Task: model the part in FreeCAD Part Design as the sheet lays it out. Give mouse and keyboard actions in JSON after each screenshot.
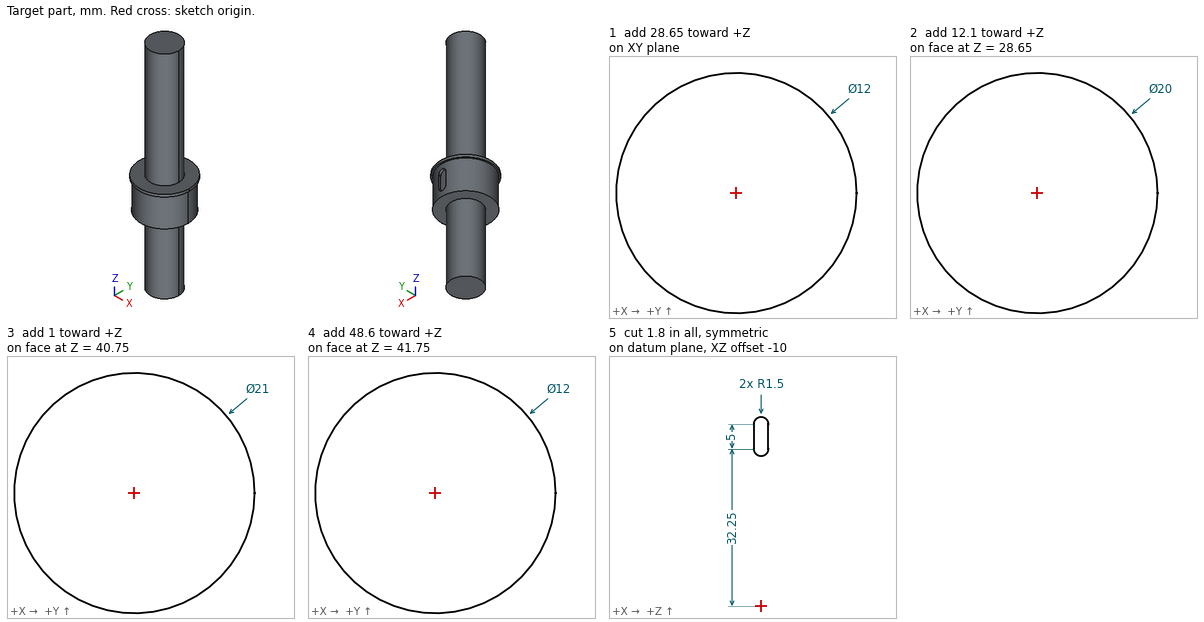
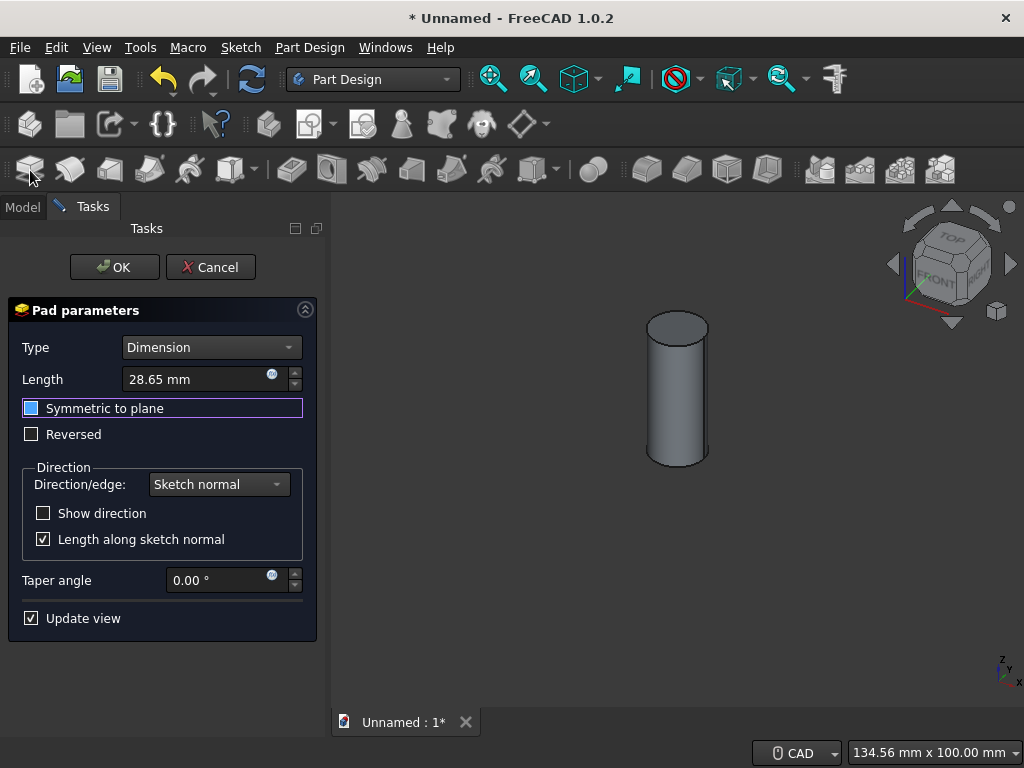
{"action": "left_click", "coordinate": [115, 267]}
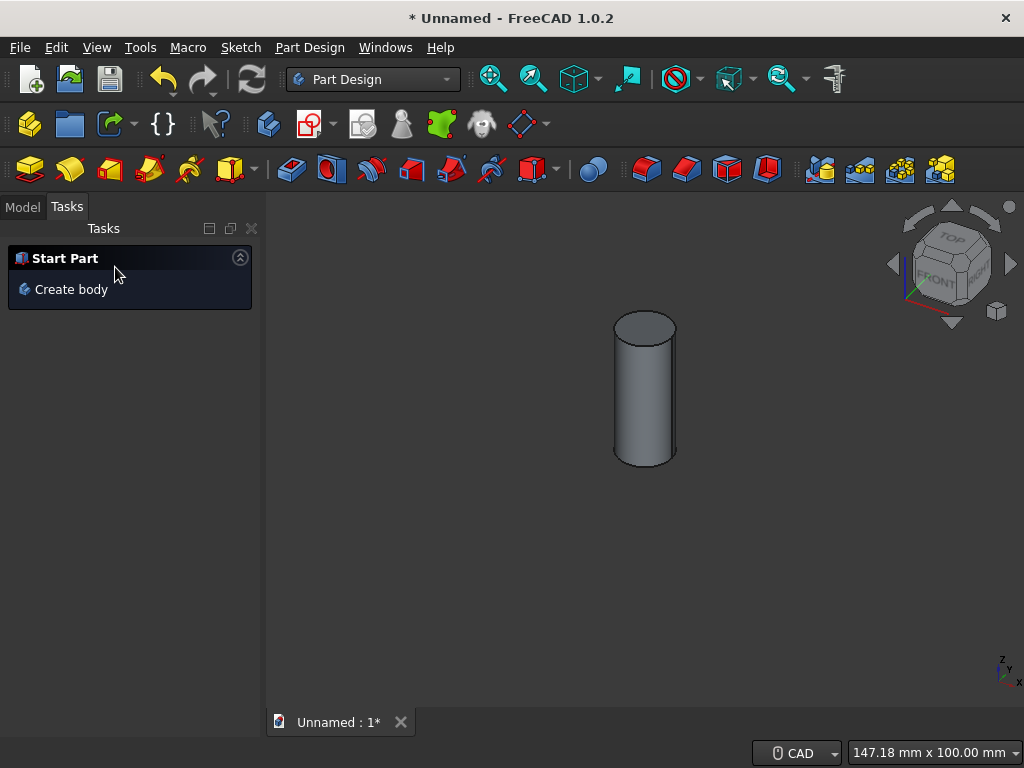
{"action": "left_click", "coordinate": [494, 80]}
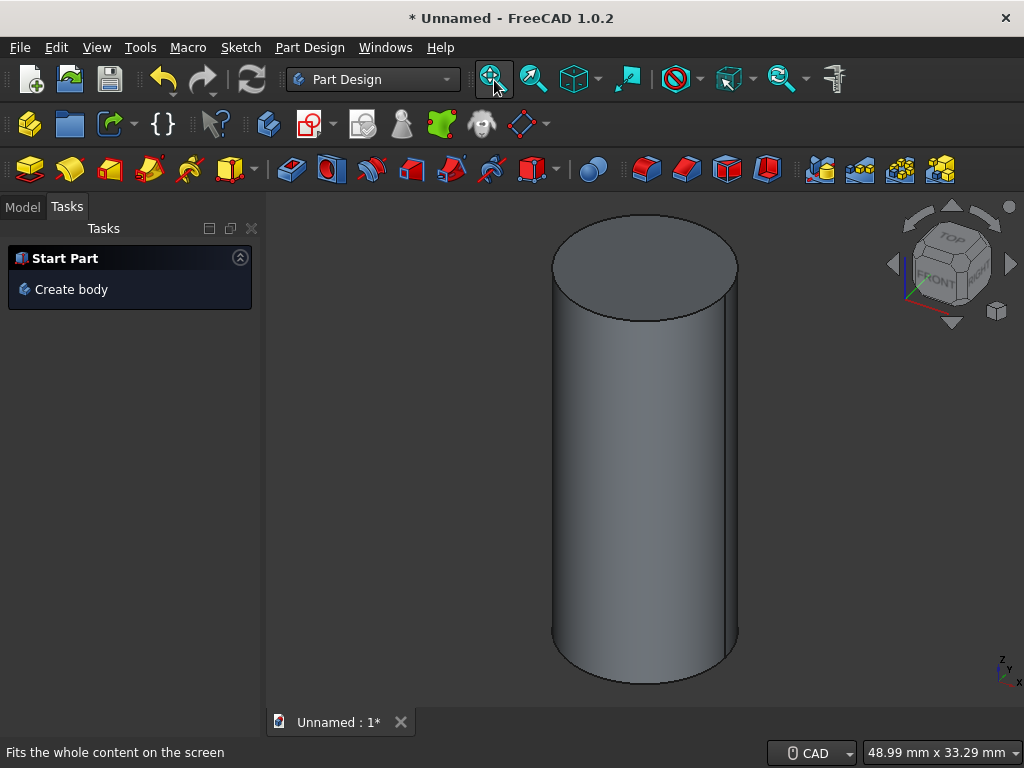
{"action": "left_click", "coordinate": [645, 267]}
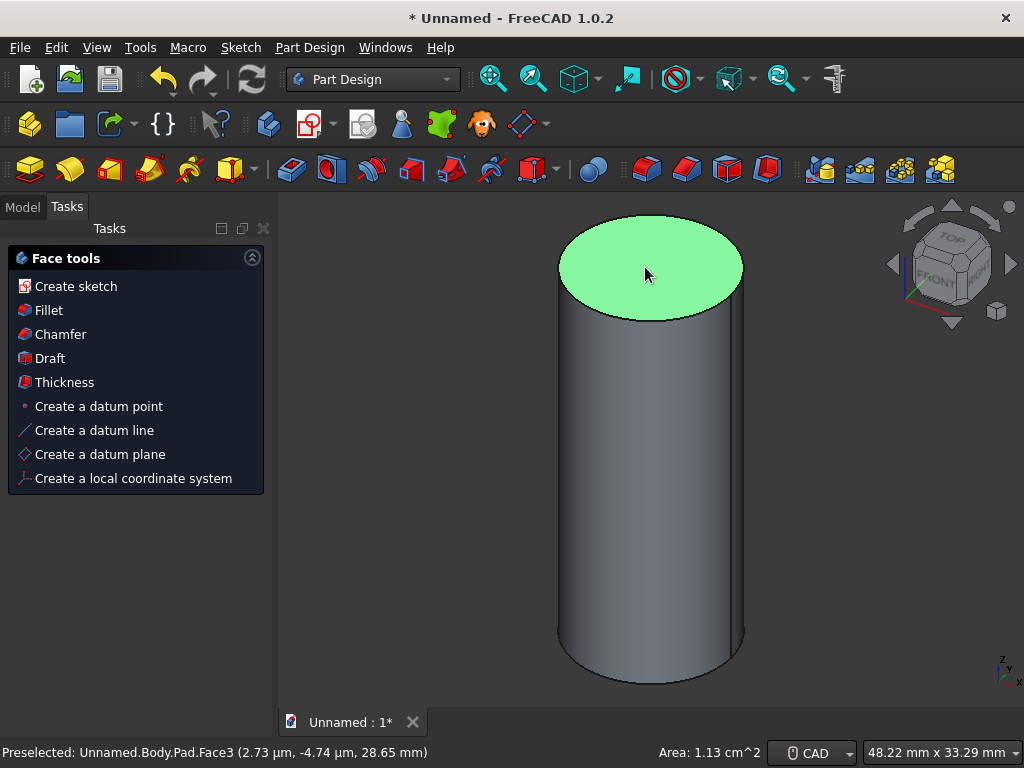
{"action": "left_click", "coordinate": [310, 124]}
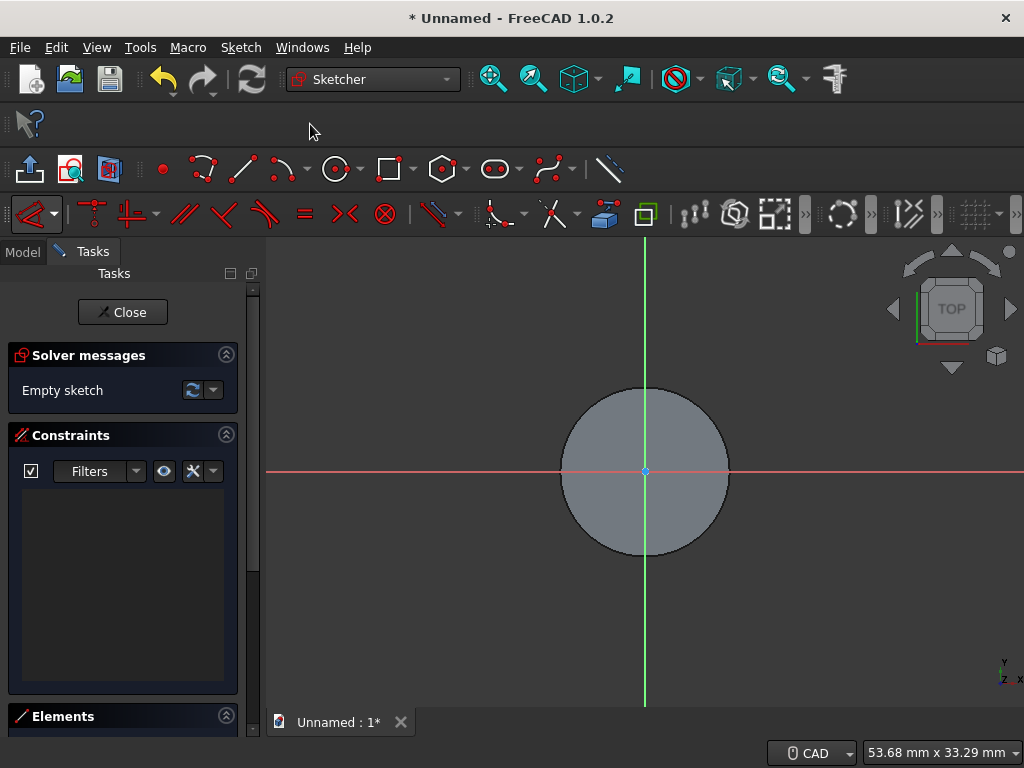
{"action": "left_click", "coordinate": [336, 170]}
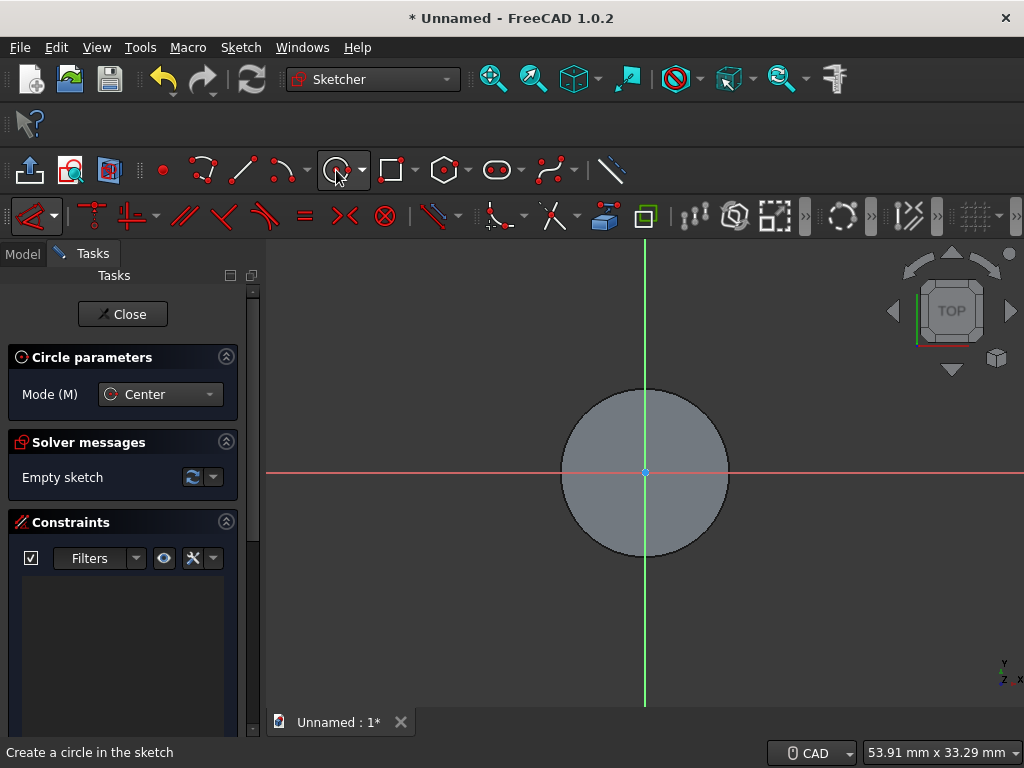
{"action": "left_click", "coordinate": [645, 473]}
{"action": "left_click", "coordinate": [744, 374]}
{"action": "key", "text": "Escape"}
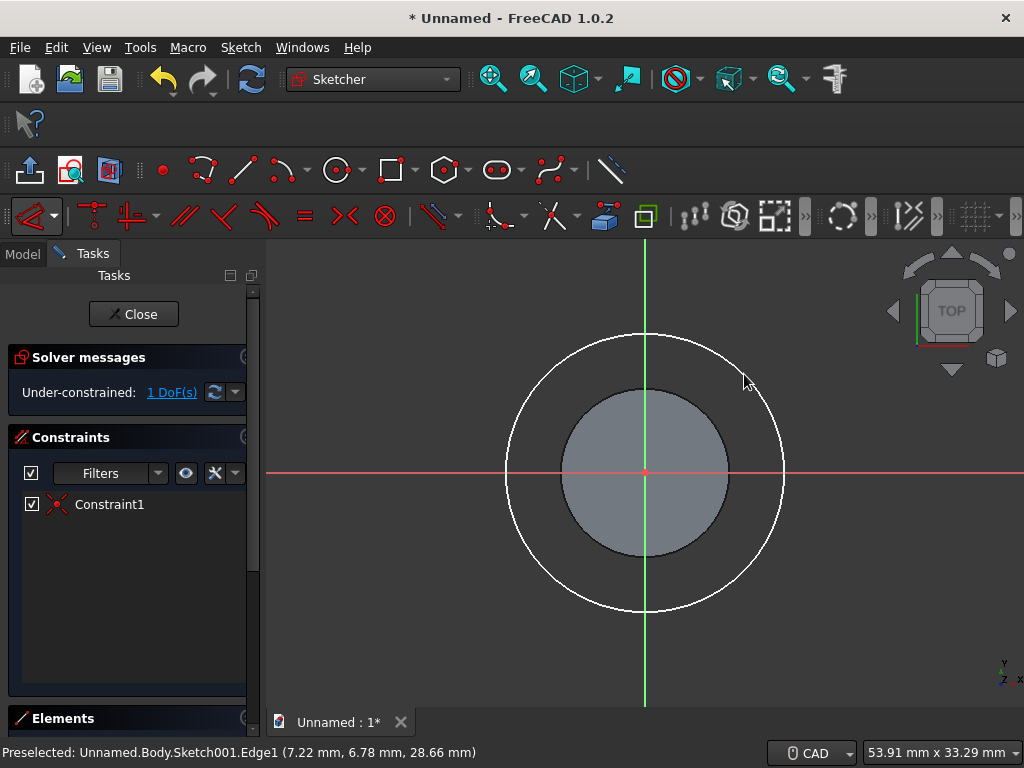
{"action": "left_click", "coordinate": [743, 374]}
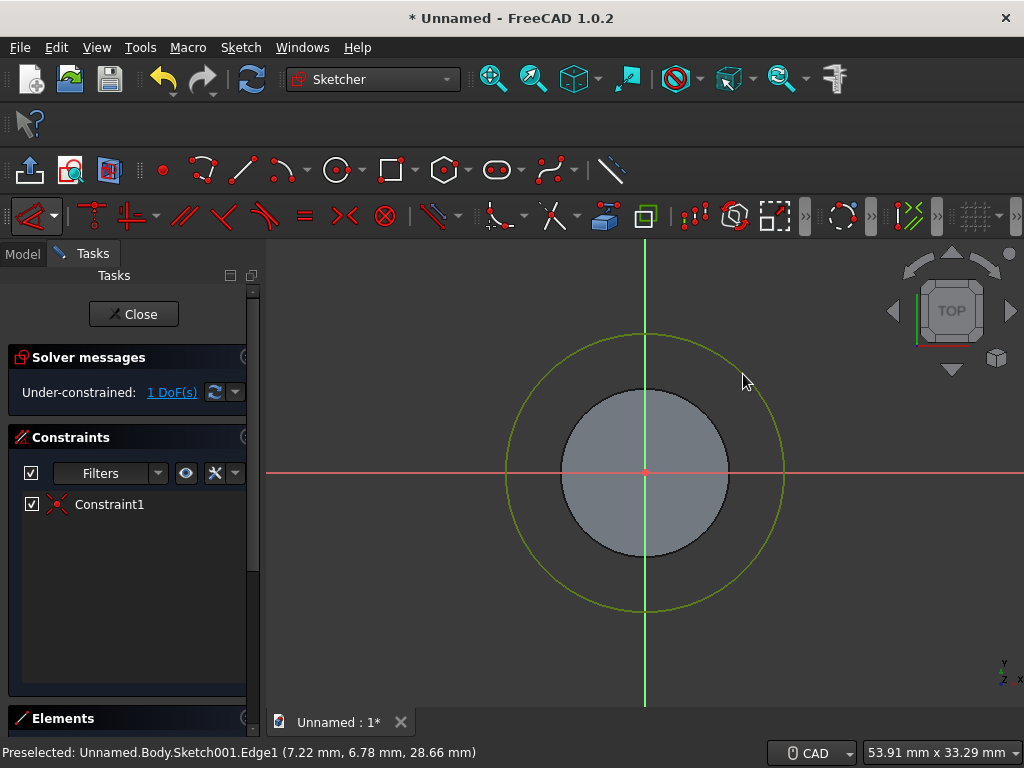
{"action": "left_click", "coordinate": [56, 216]}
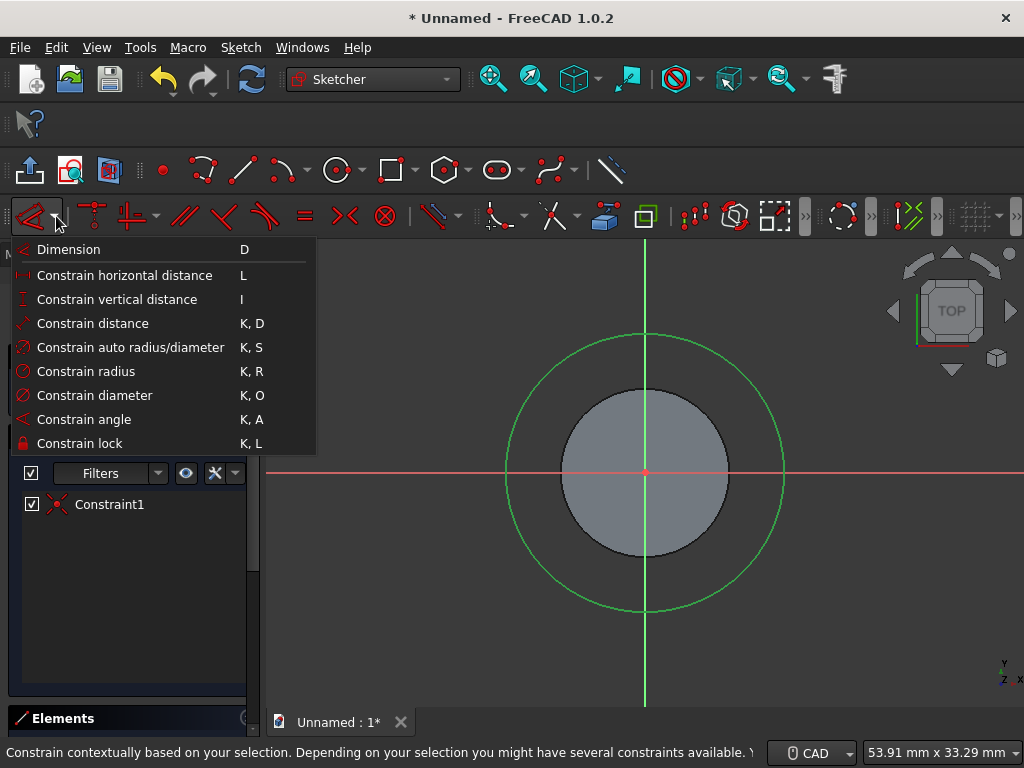
{"action": "left_click", "coordinate": [164, 395]}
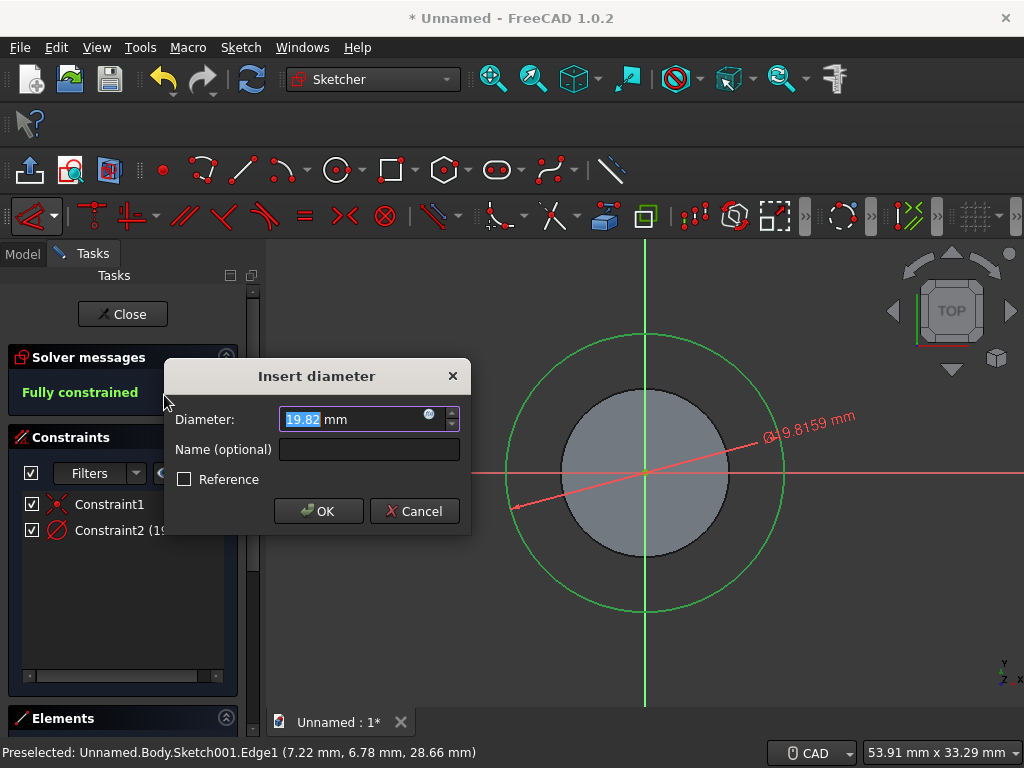
{"action": "type", "text": "20"}
{"action": "key", "text": "Return"}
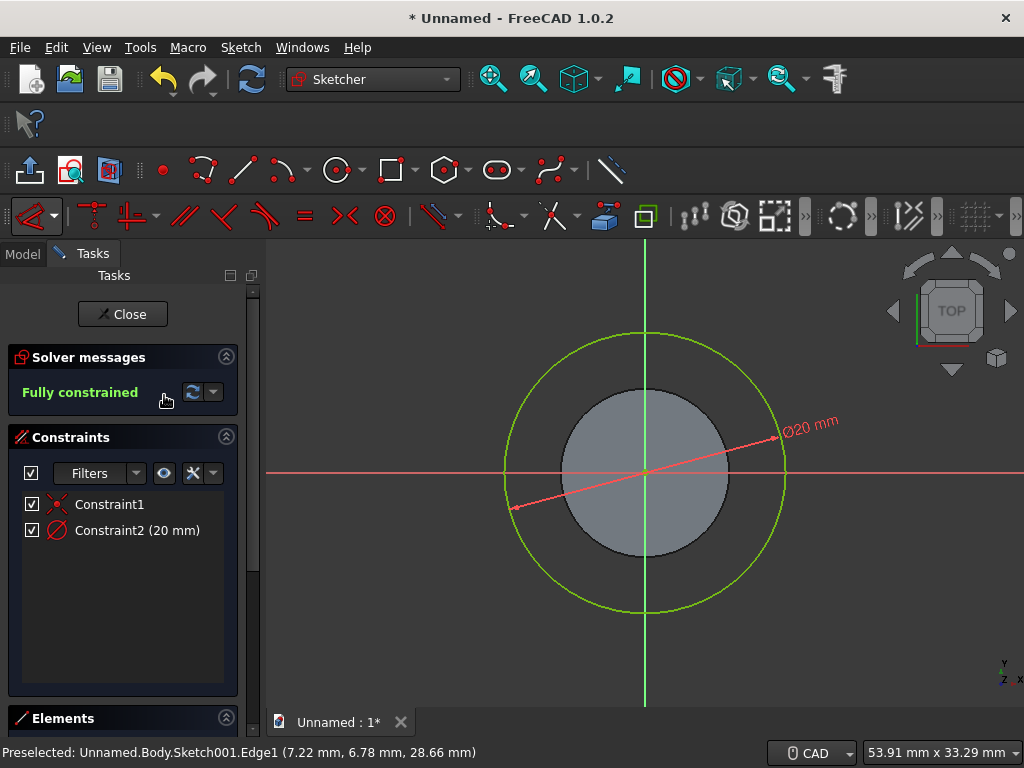
{"action": "left_click", "coordinate": [123, 314]}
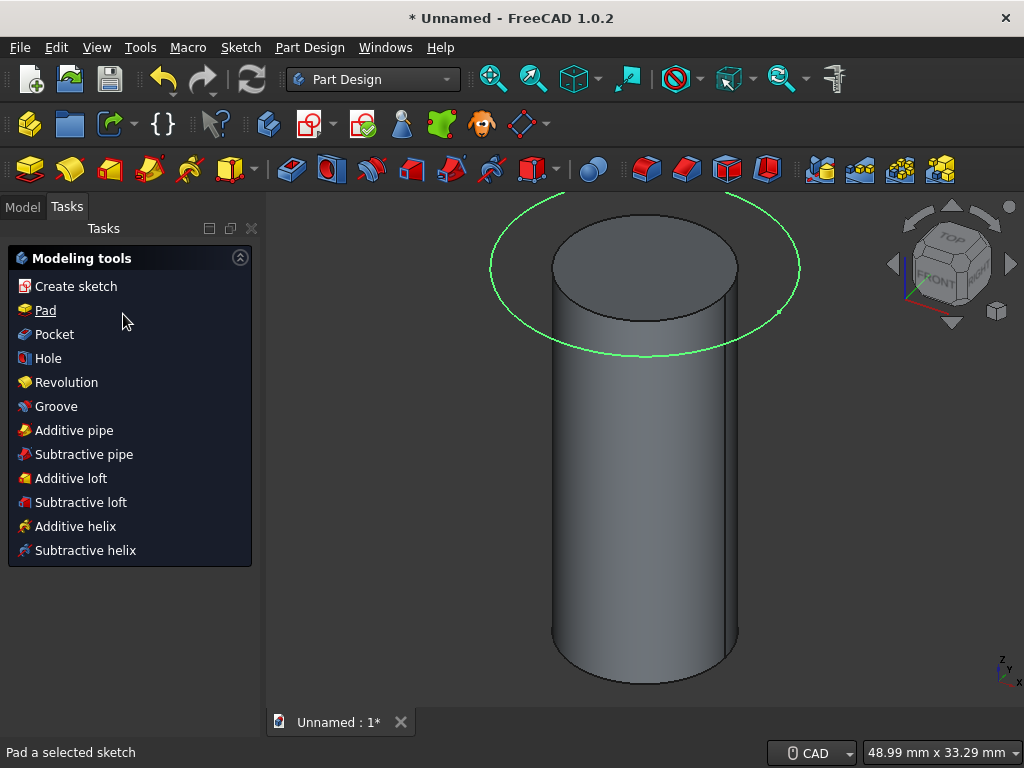
{"action": "left_click", "coordinate": [30, 170]}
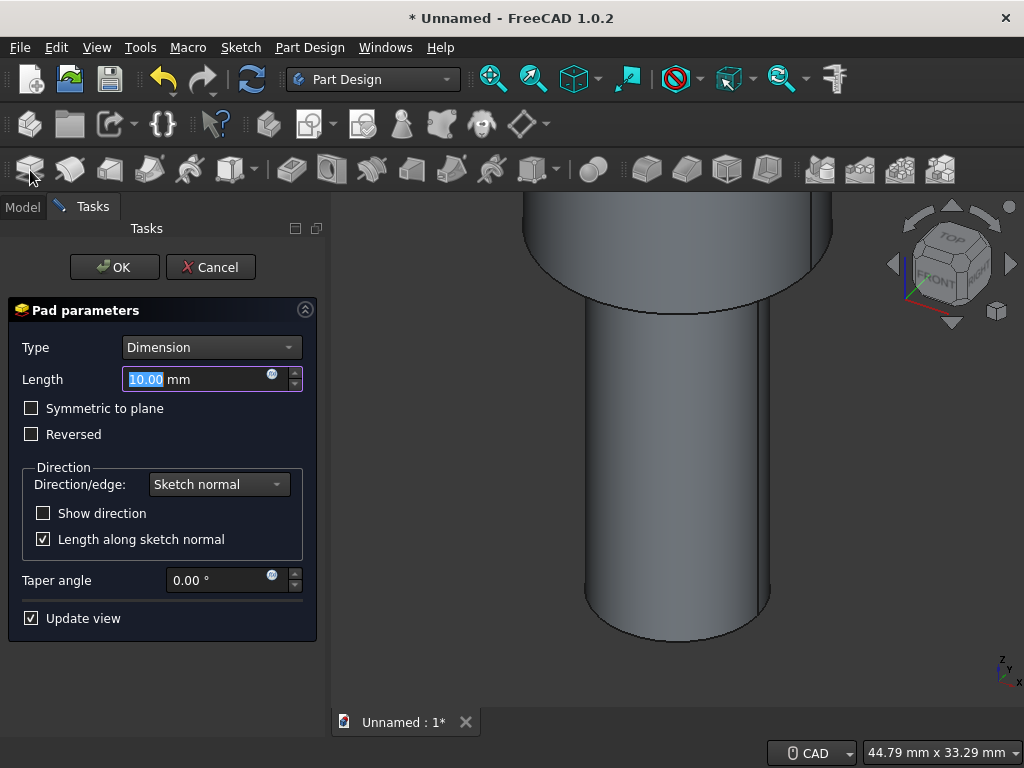
{"action": "type", "text": "12.1"}
{"action": "key", "text": "Tab"}